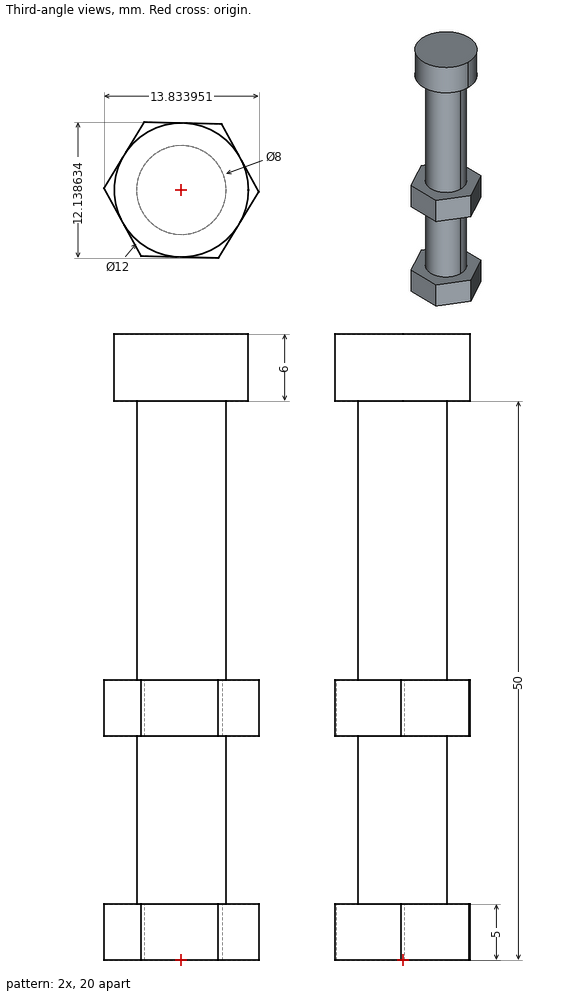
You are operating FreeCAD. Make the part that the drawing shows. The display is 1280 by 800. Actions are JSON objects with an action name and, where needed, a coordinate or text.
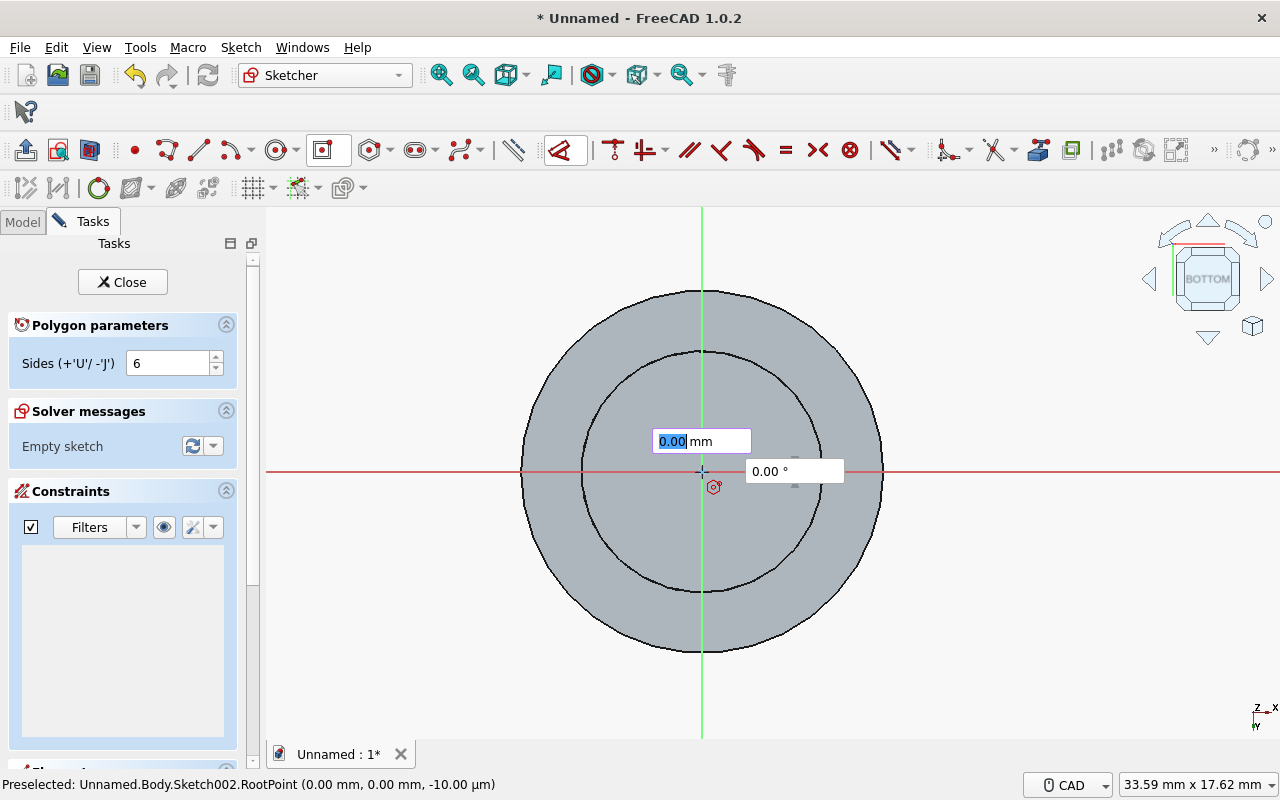
{"action": "left_click", "coordinate": [811, 650]}
{"action": "key", "text": "Escape"}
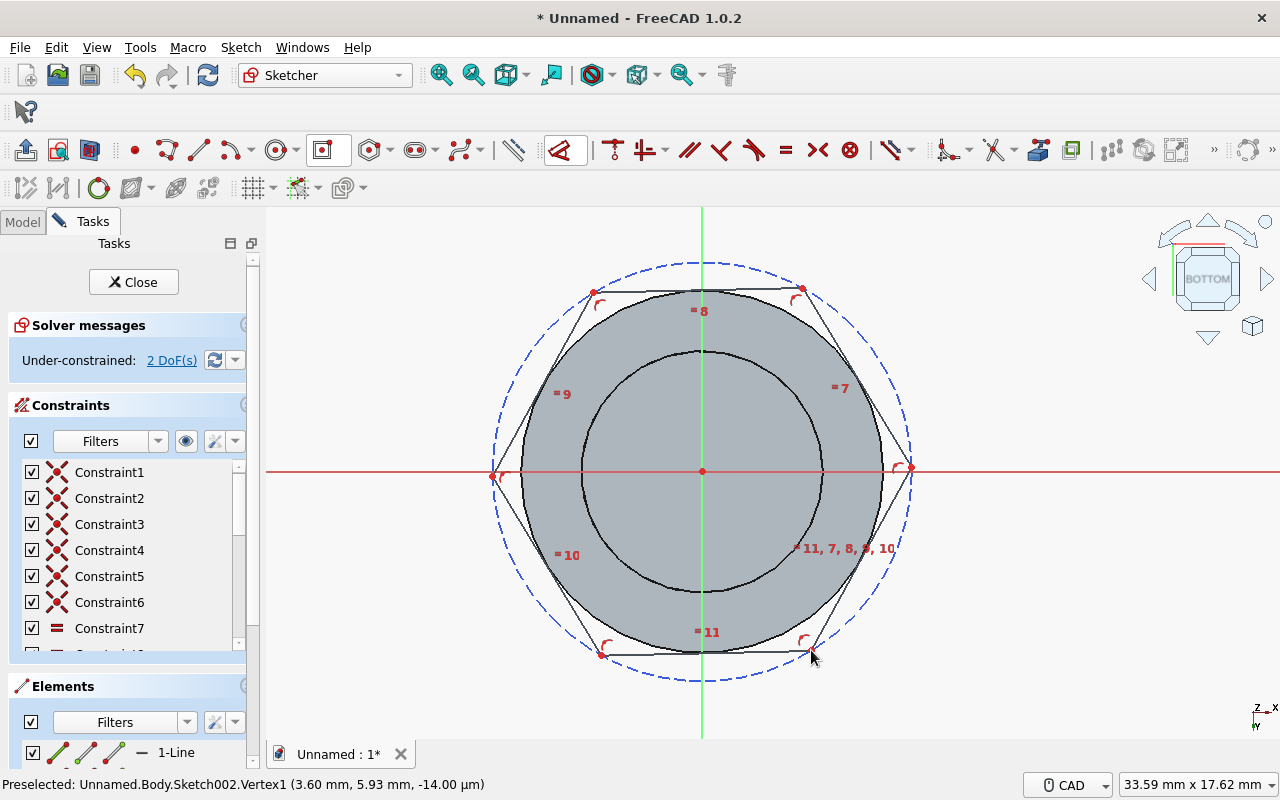
{"action": "left_click", "coordinate": [560, 150]}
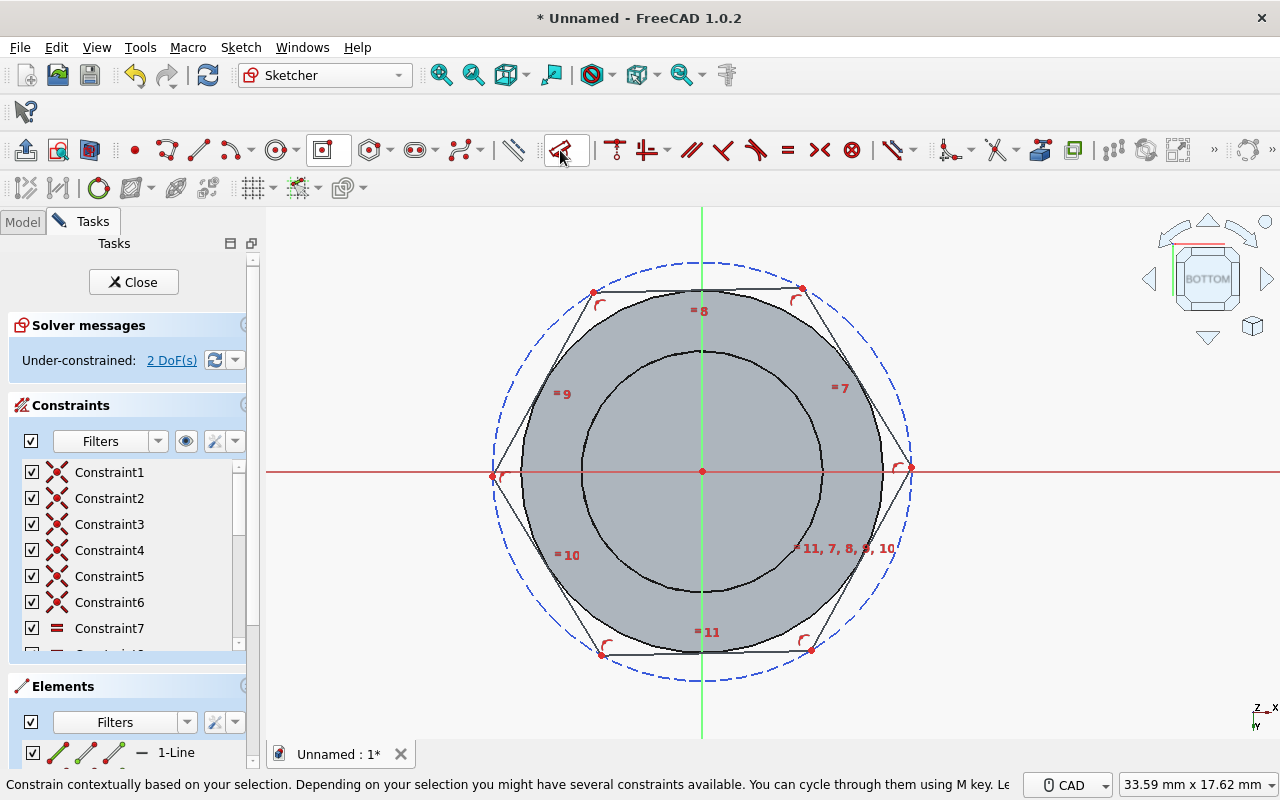
{"action": "left_click", "coordinate": [493, 477]}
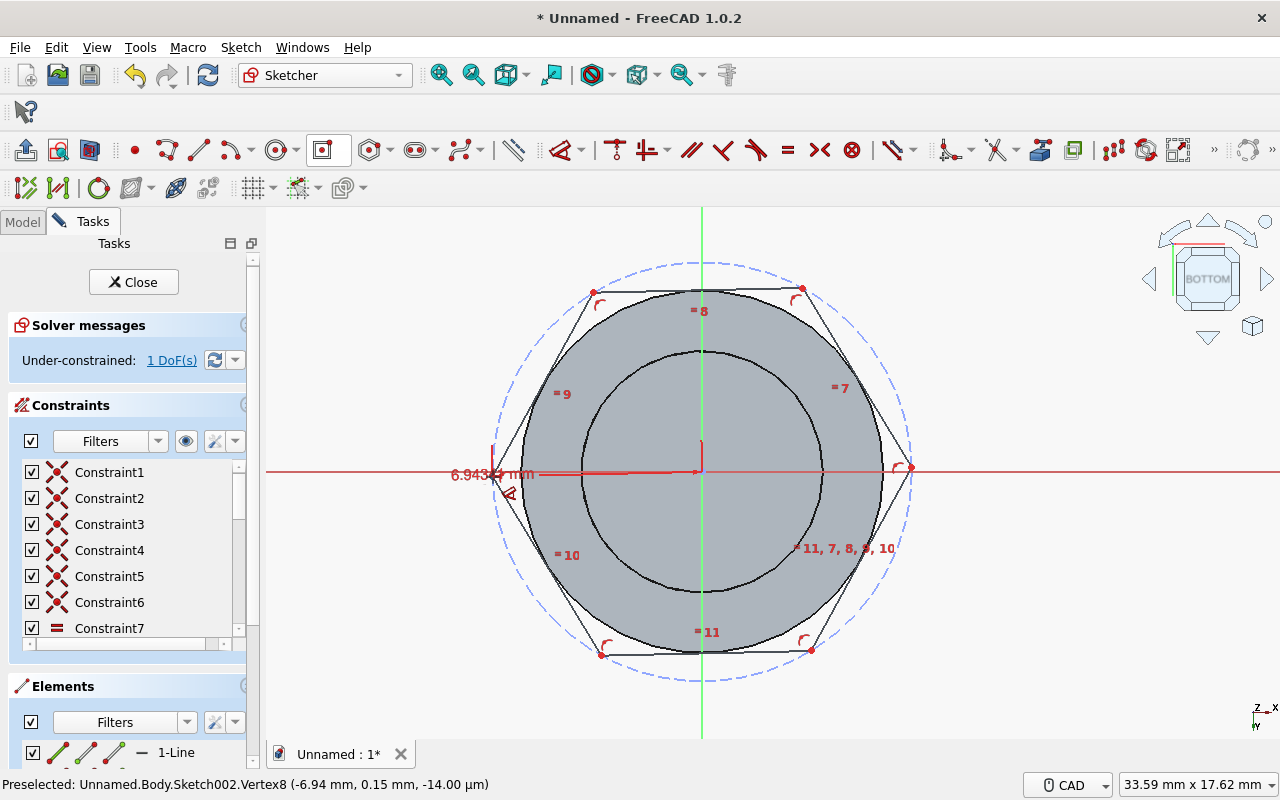
{"action": "left_click", "coordinate": [912, 467]}
{"action": "left_click", "coordinate": [606, 433]}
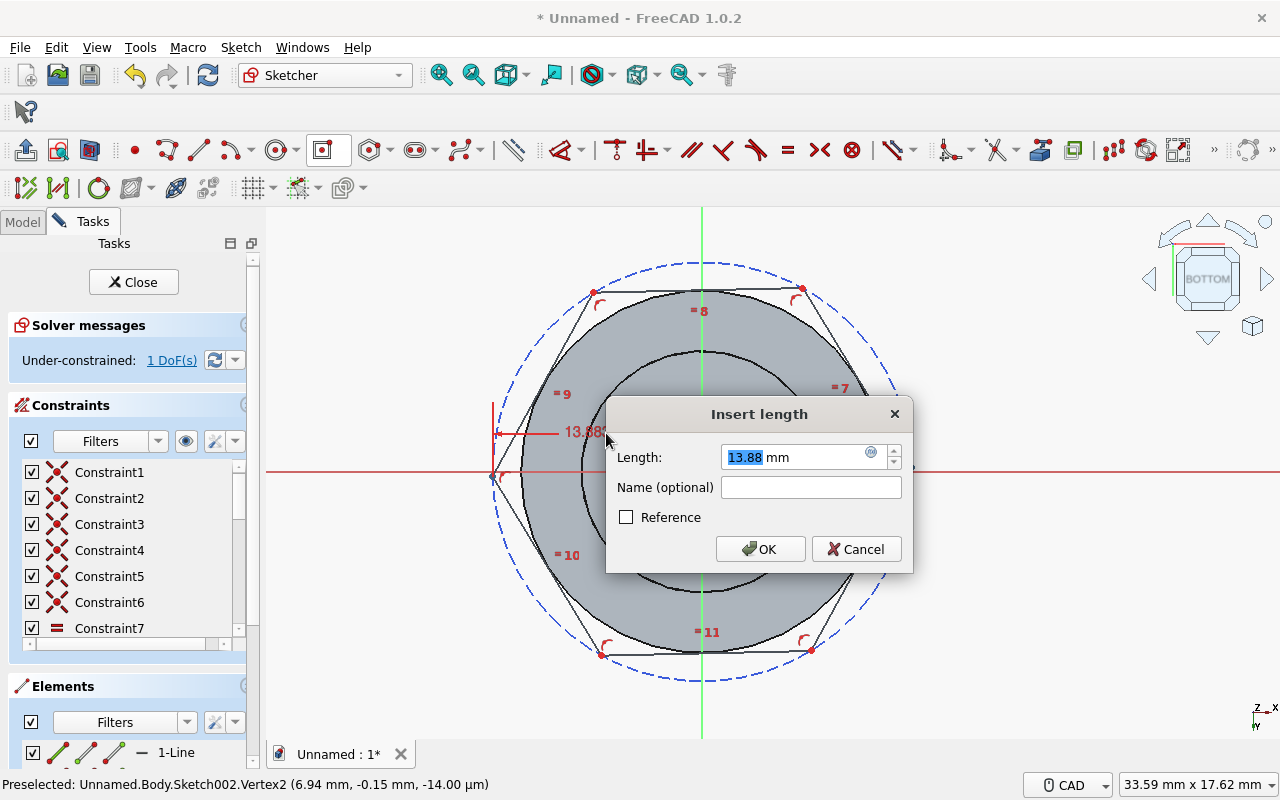
{"action": "type", "text": "13.833951"}
{"action": "key", "text": "Return"}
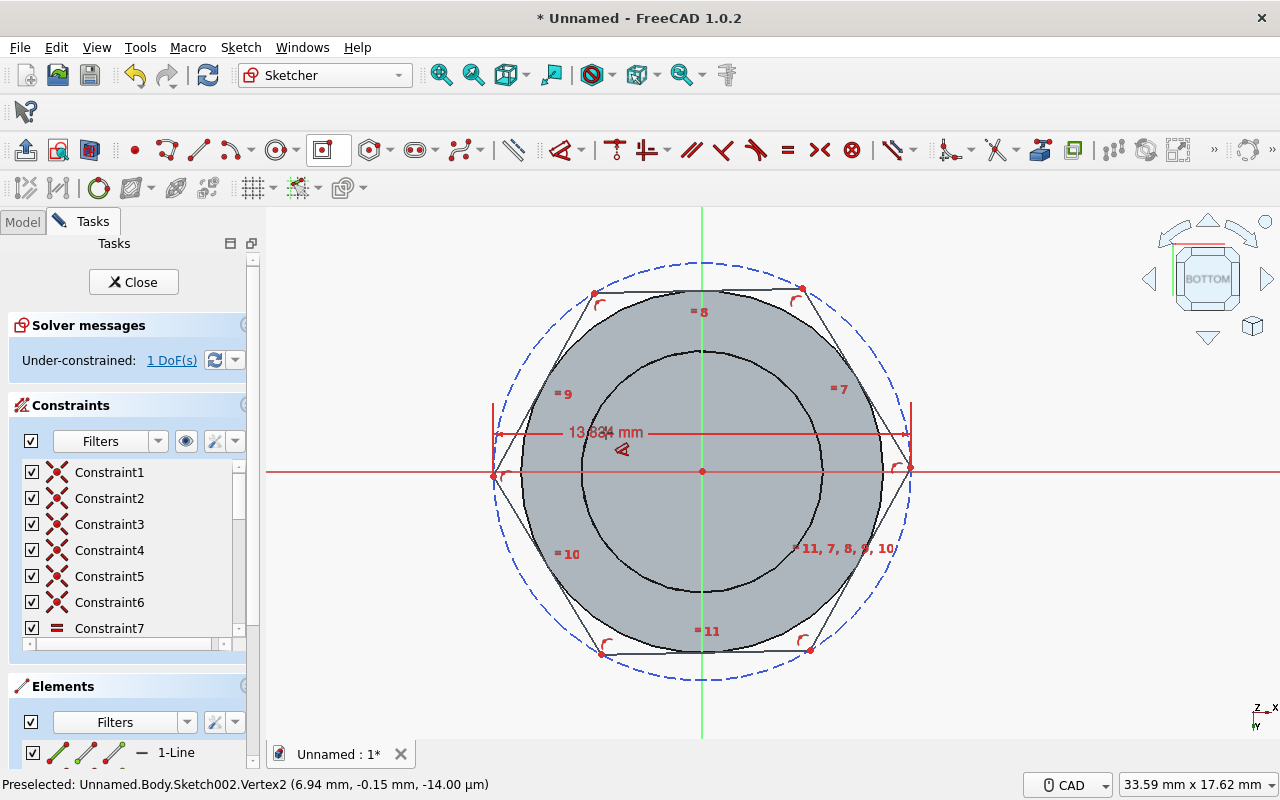
{"action": "left_click", "coordinate": [601, 655]}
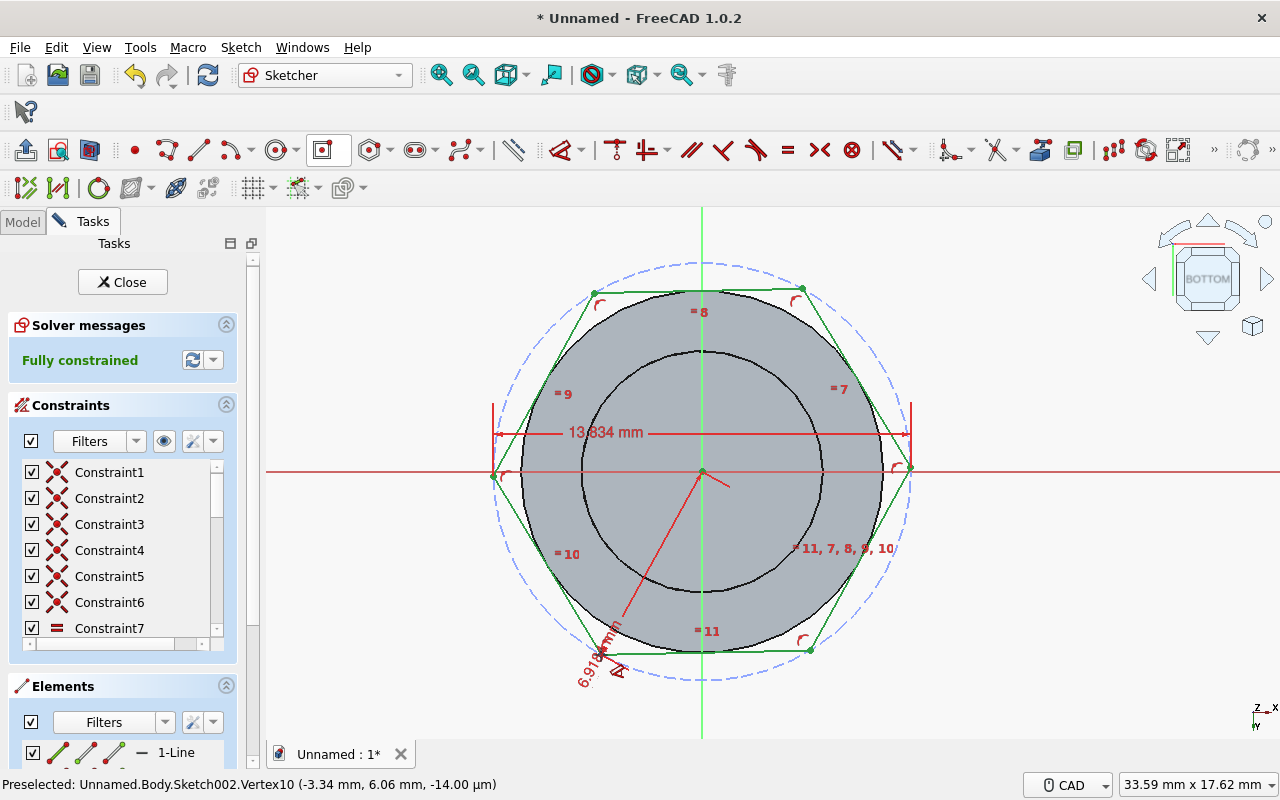
{"action": "left_click", "coordinate": [803, 289]}
{"action": "left_click", "coordinate": [837, 388]}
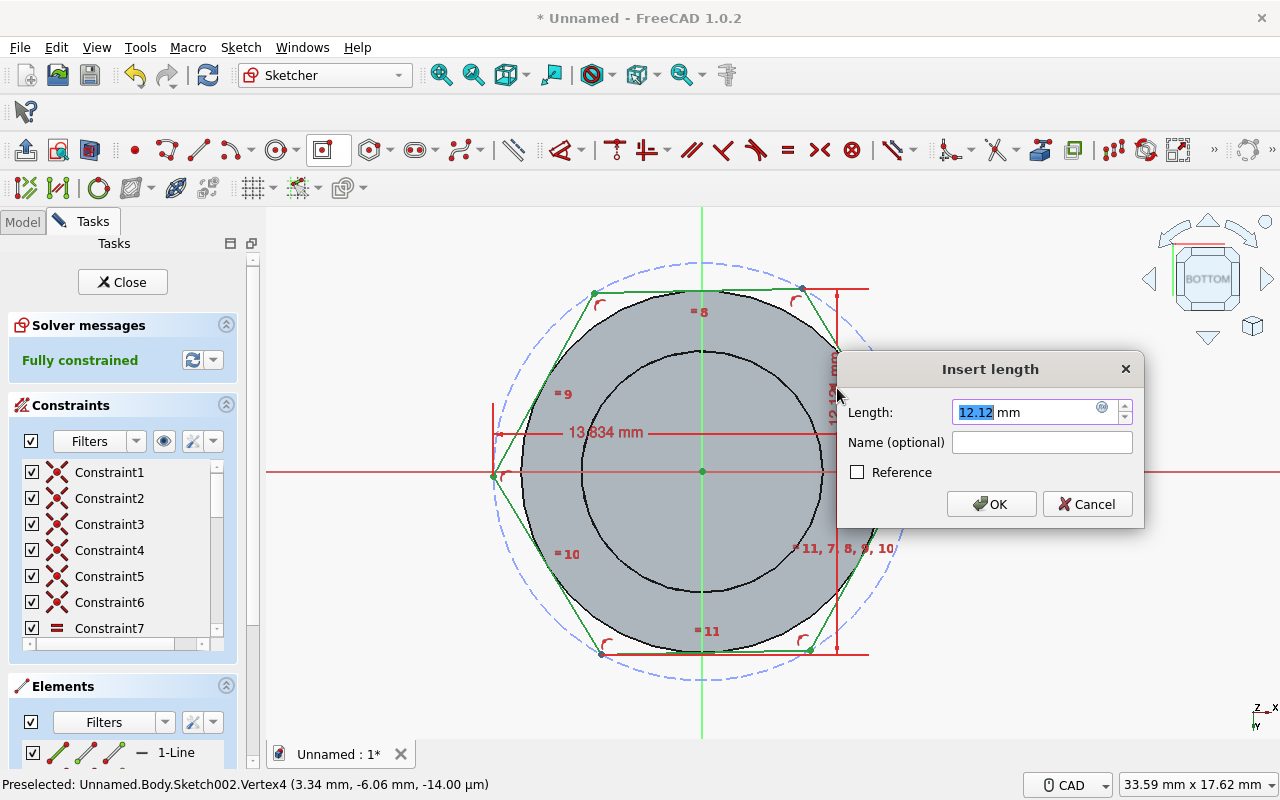
{"action": "type", "text": "12.138634"}
{"action": "key", "text": "Return"}
{"action": "key", "text": "Escape"}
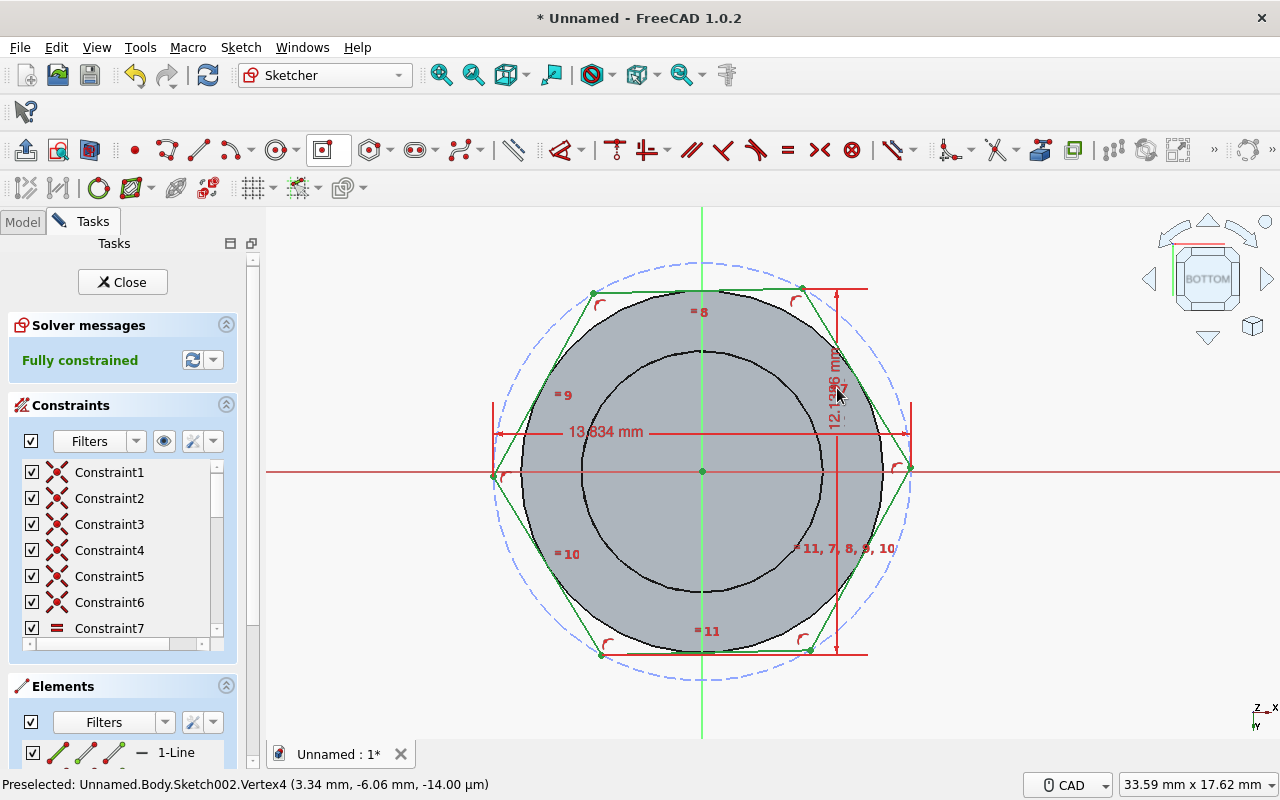
{"action": "left_click", "coordinate": [123, 282]}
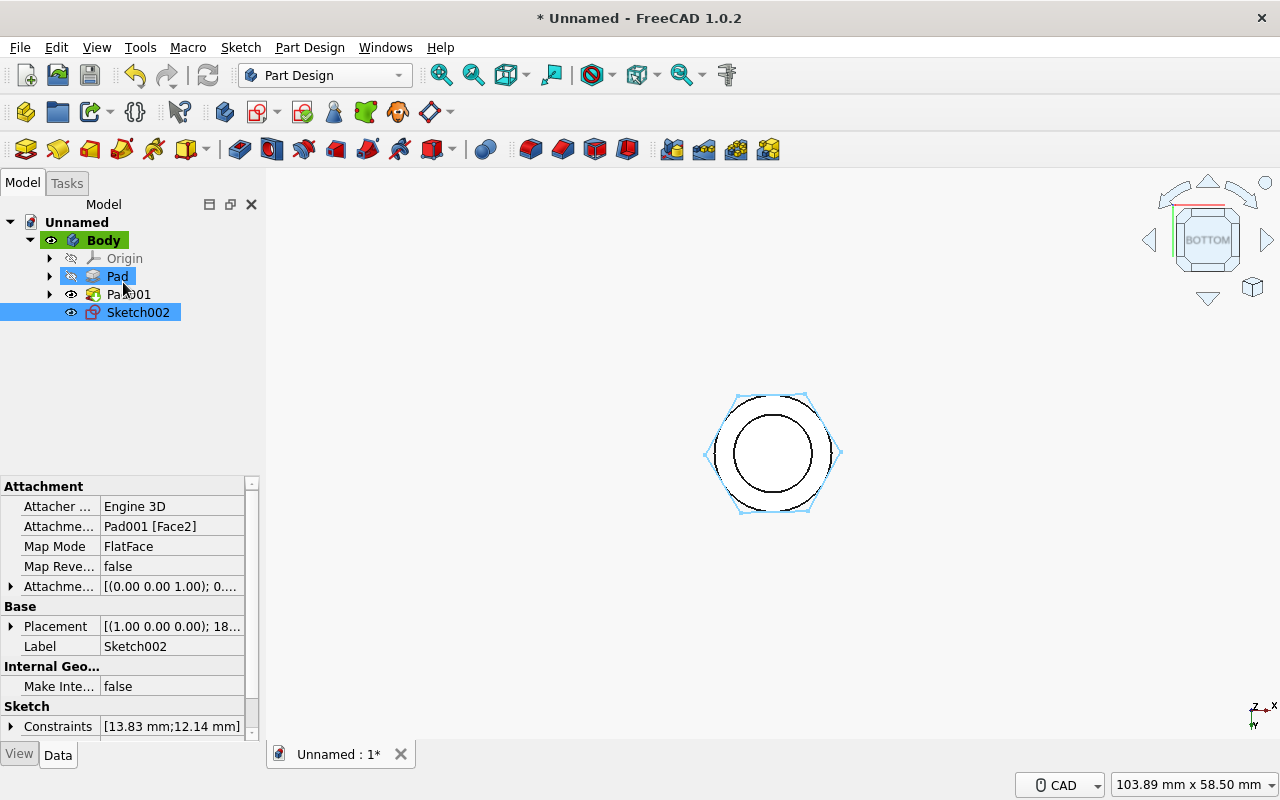
{"action": "left_click", "coordinate": [26, 150]}